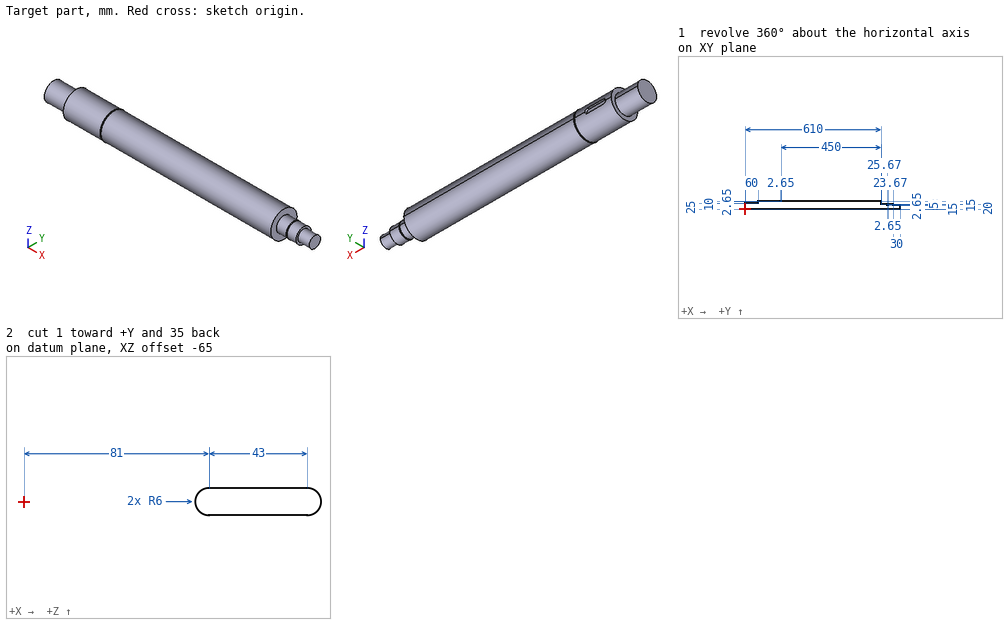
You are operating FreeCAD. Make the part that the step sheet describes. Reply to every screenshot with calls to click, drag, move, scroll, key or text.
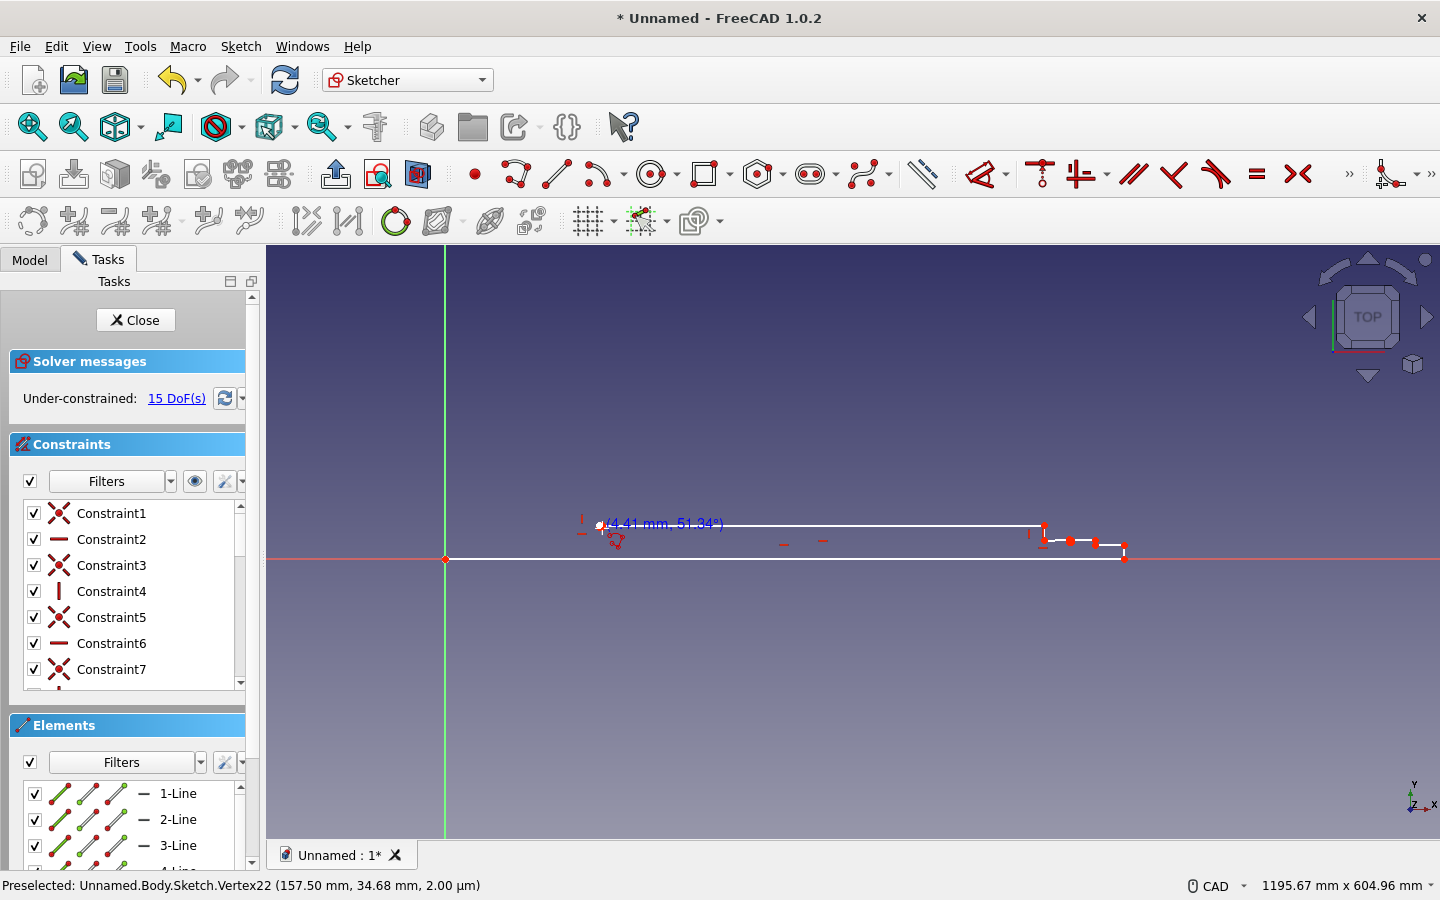
click(504, 525)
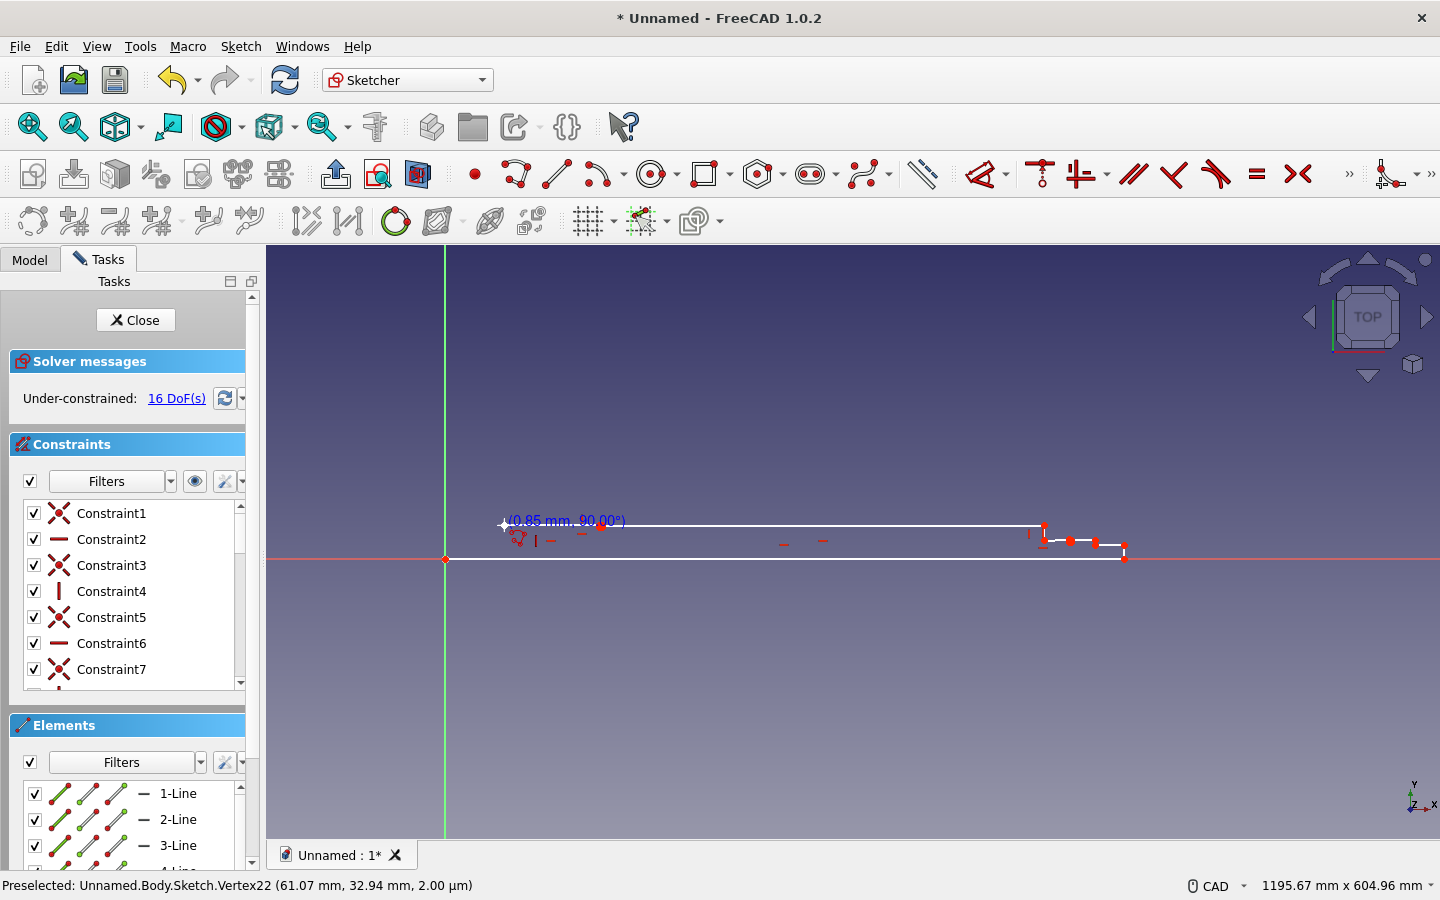
scroll(504, 535, up, 3)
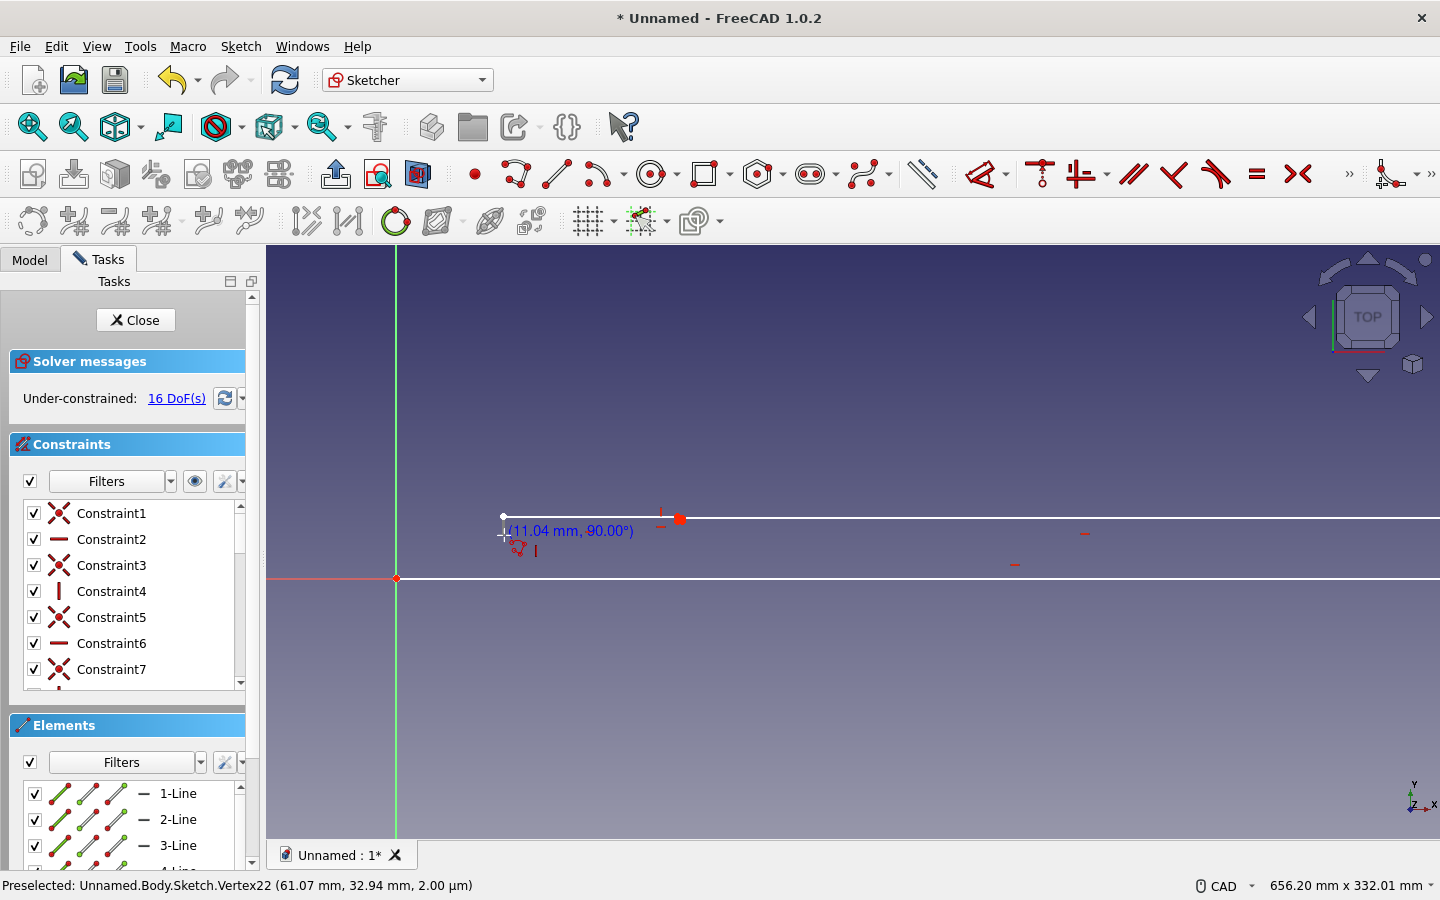
click(504, 534)
click(405, 534)
click(396, 579)
key(Escape)
key(Escape)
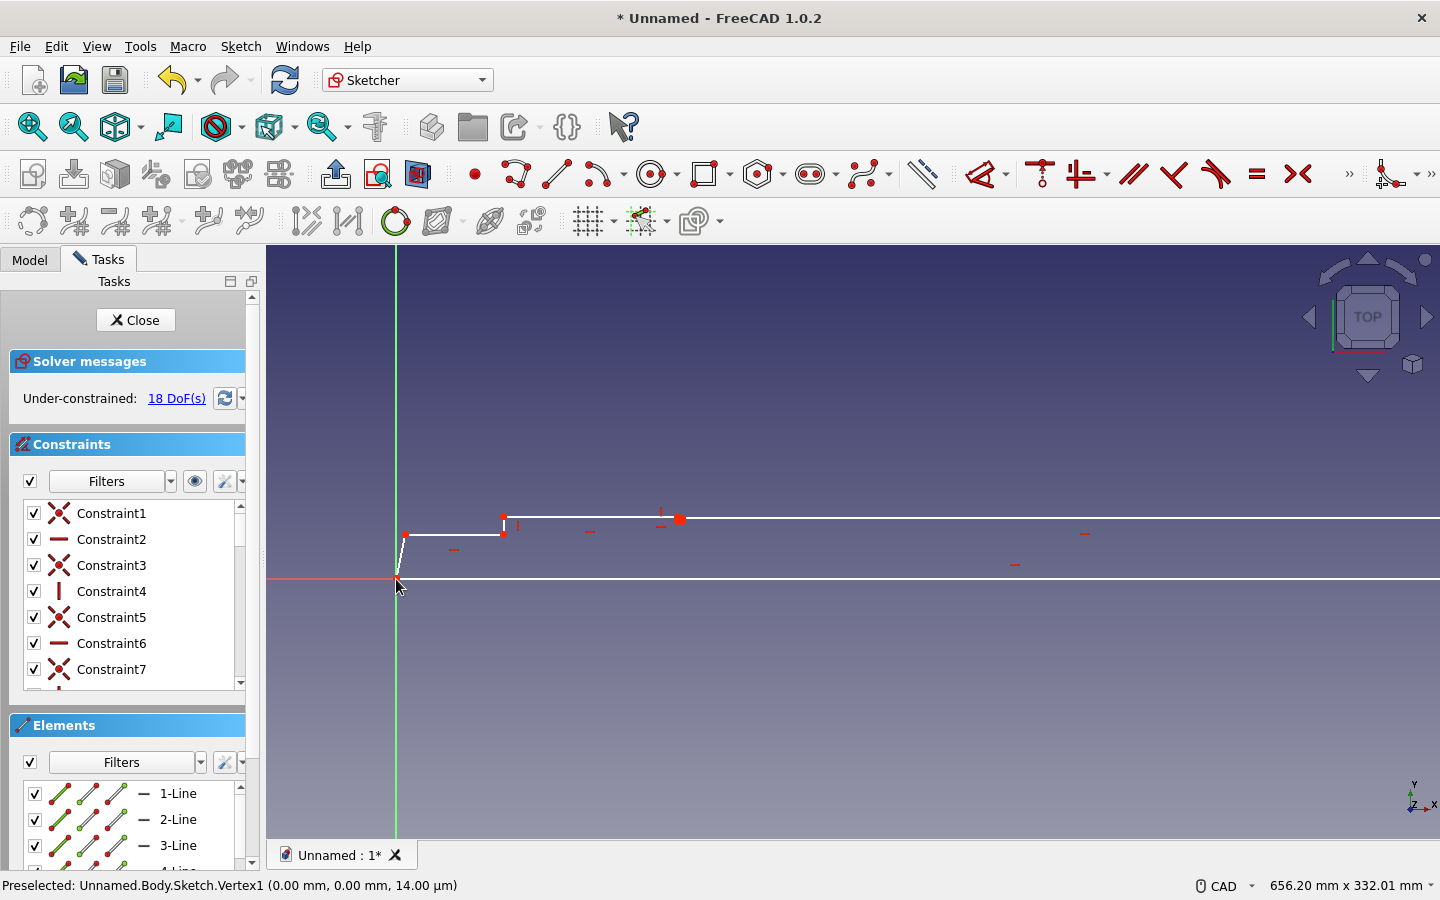
scroll(504, 535, down, 3)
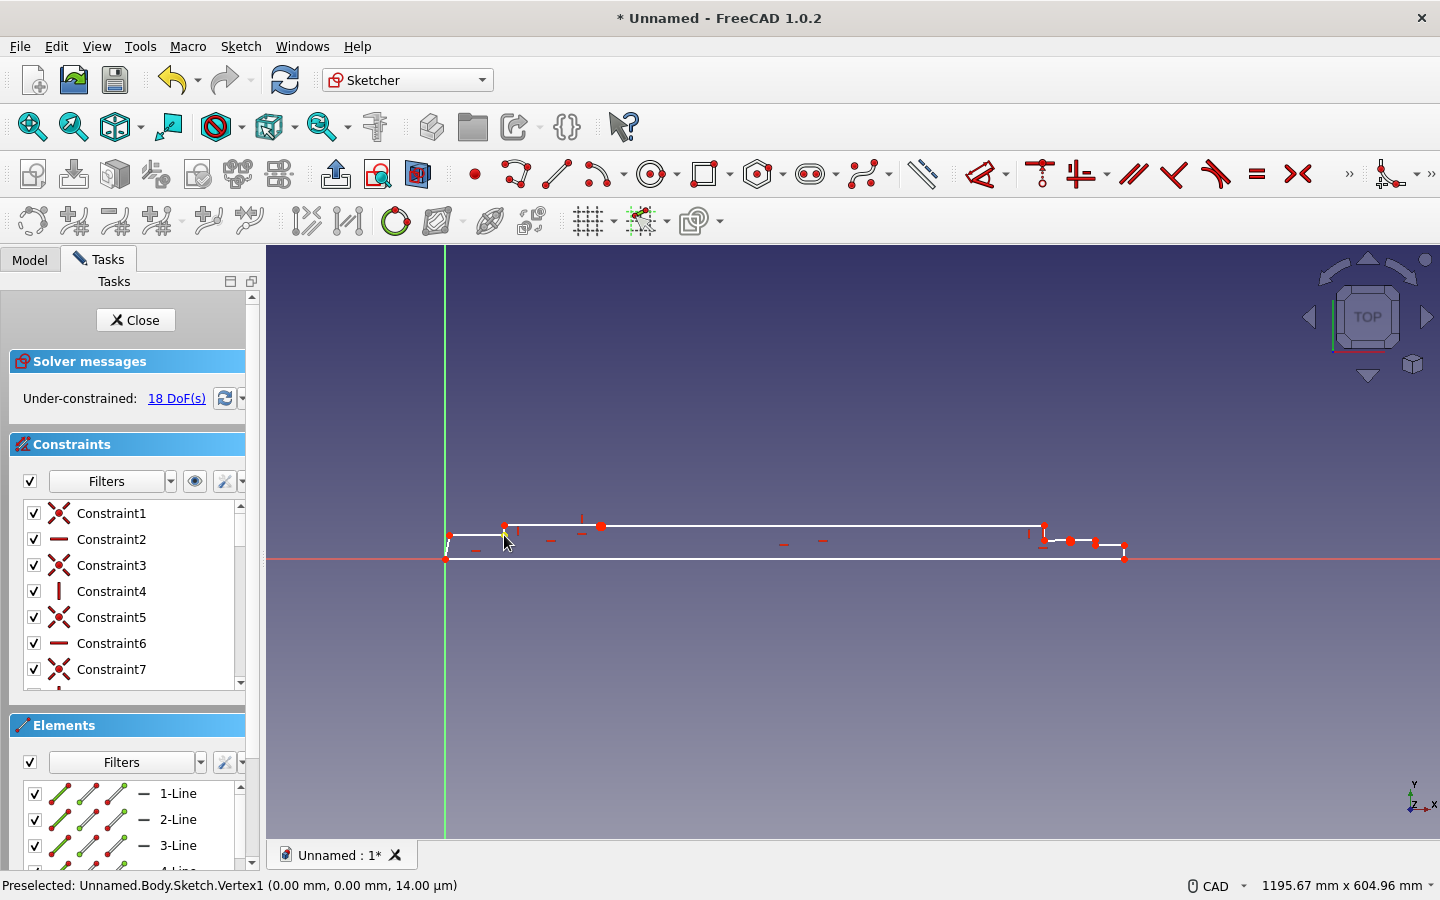
scroll(1062, 540, up, 4)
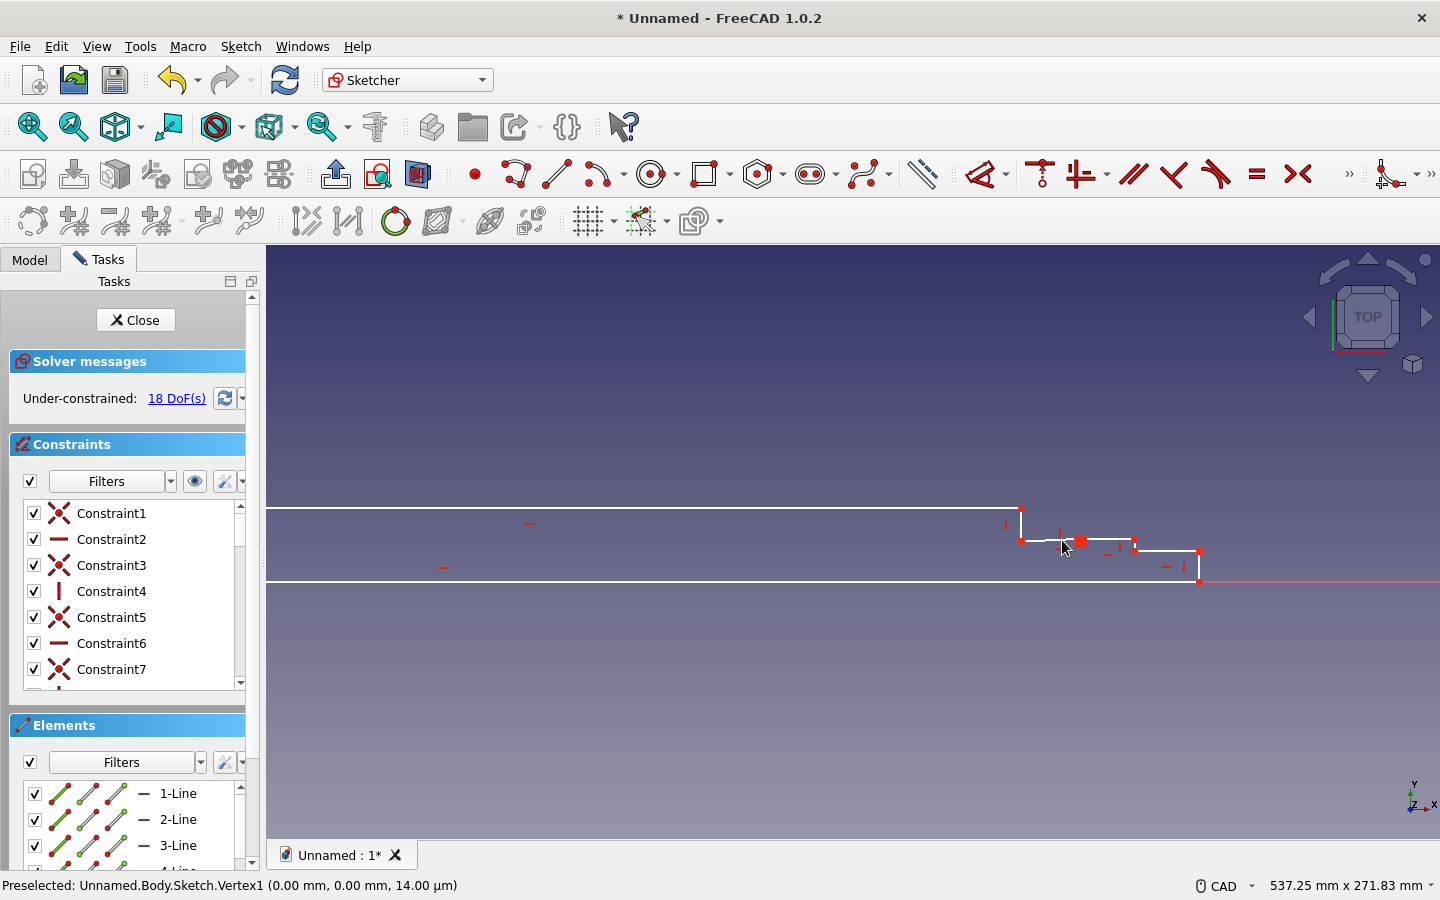
click(1038, 541)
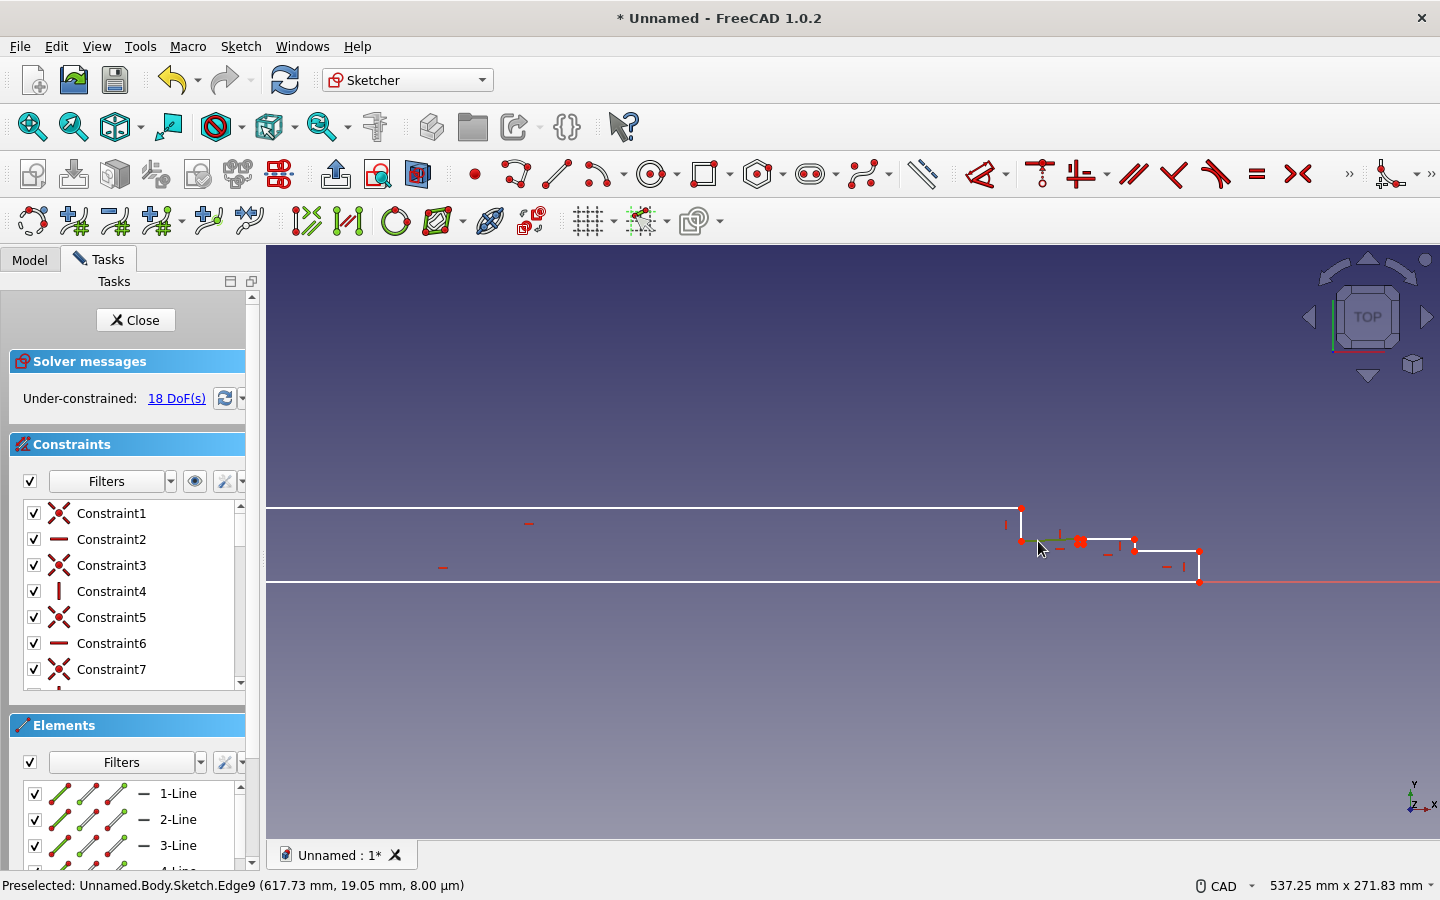
key(h)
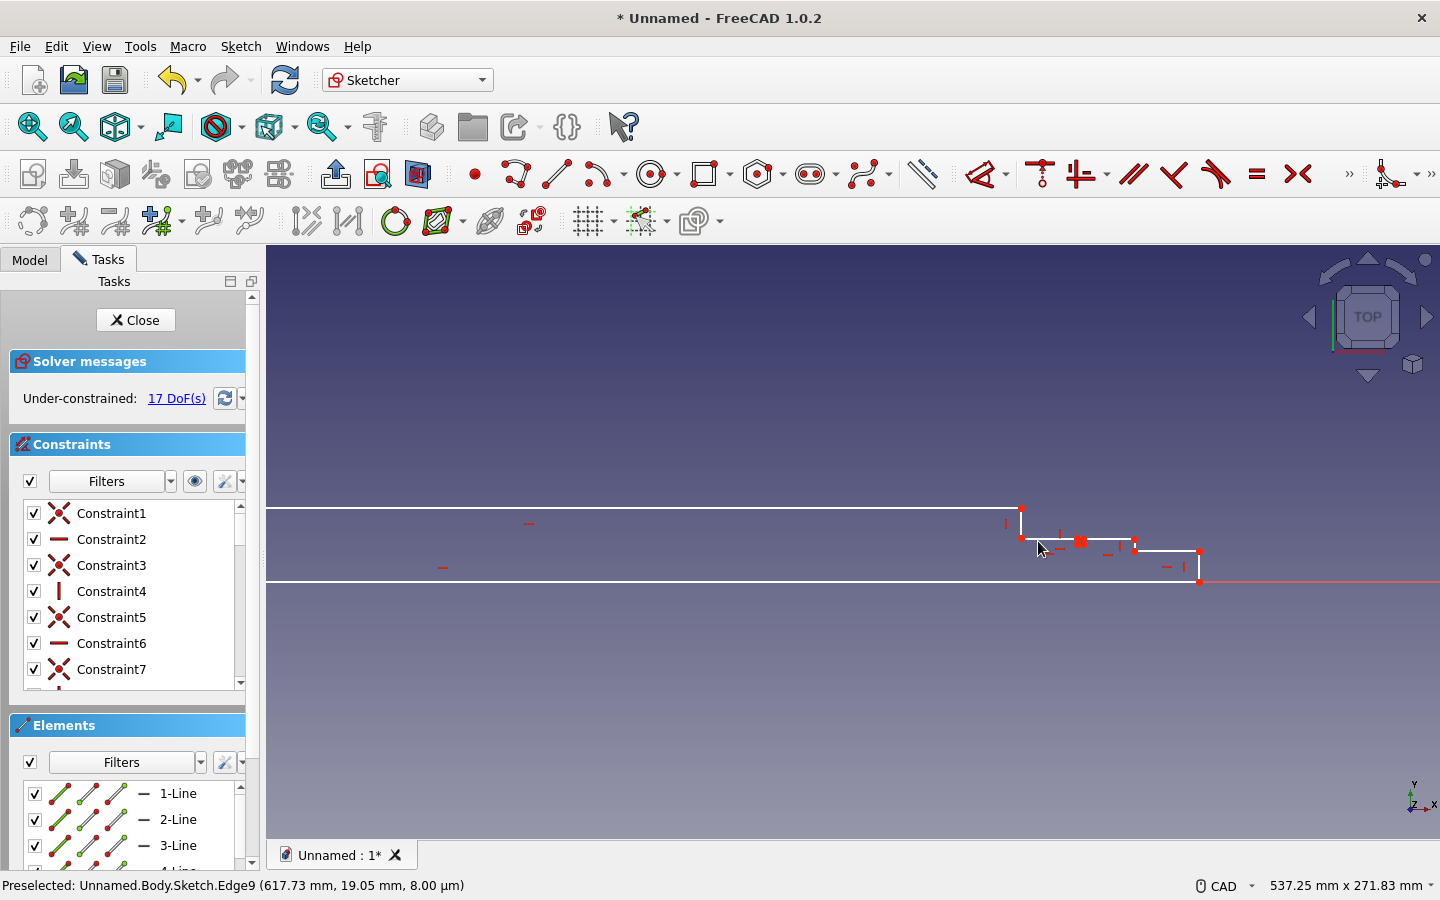
scroll(1062, 540, down, 4)